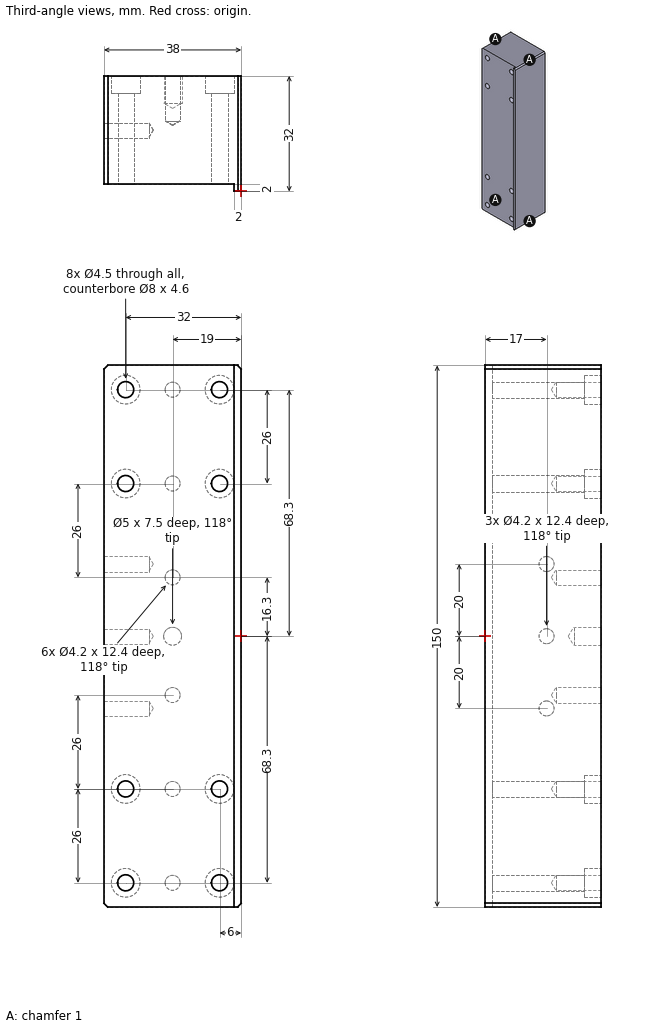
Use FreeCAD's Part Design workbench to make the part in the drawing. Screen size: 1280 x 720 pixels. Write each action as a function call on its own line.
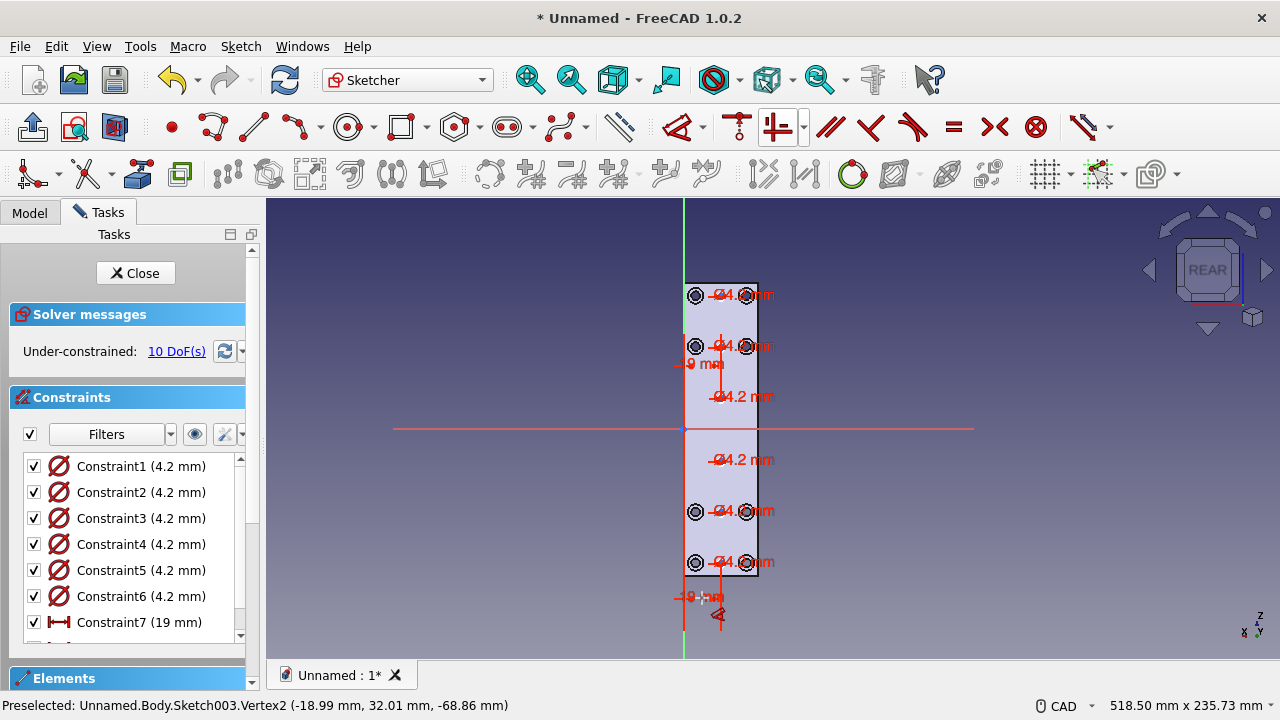
click(721, 513)
click(702, 547)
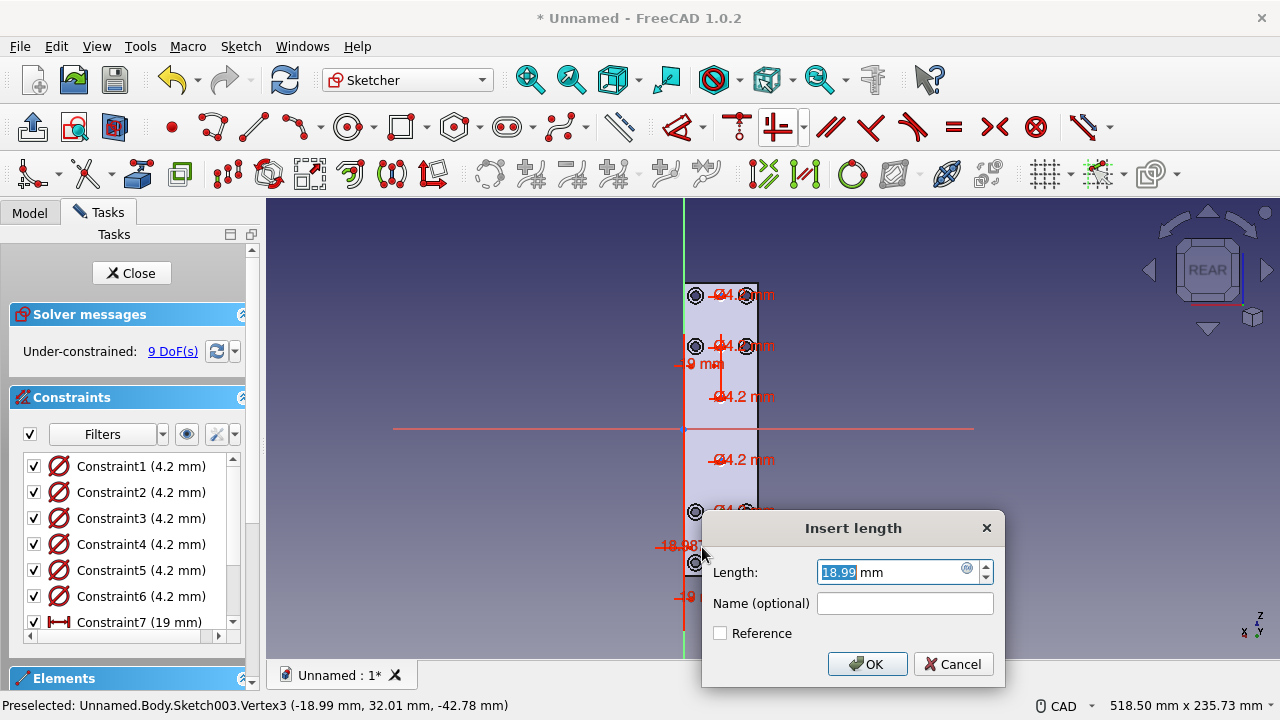
text(19)
key(Return)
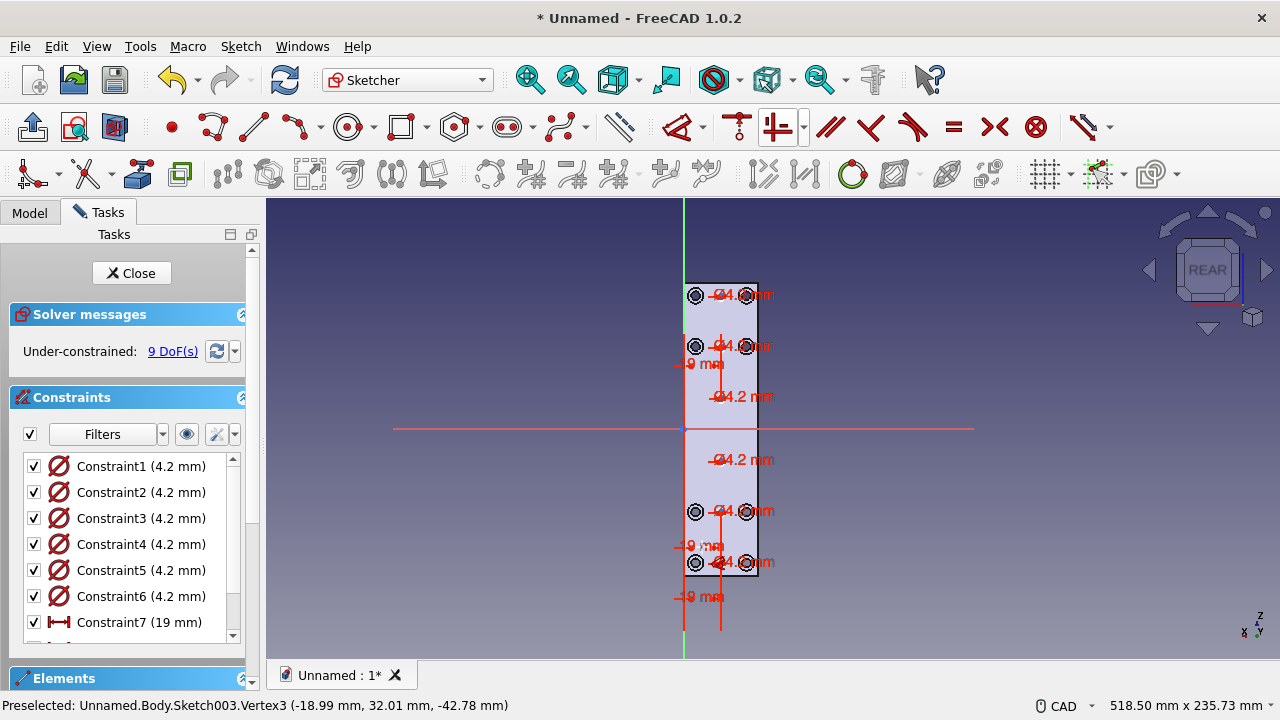
click(721, 348)
click(702, 314)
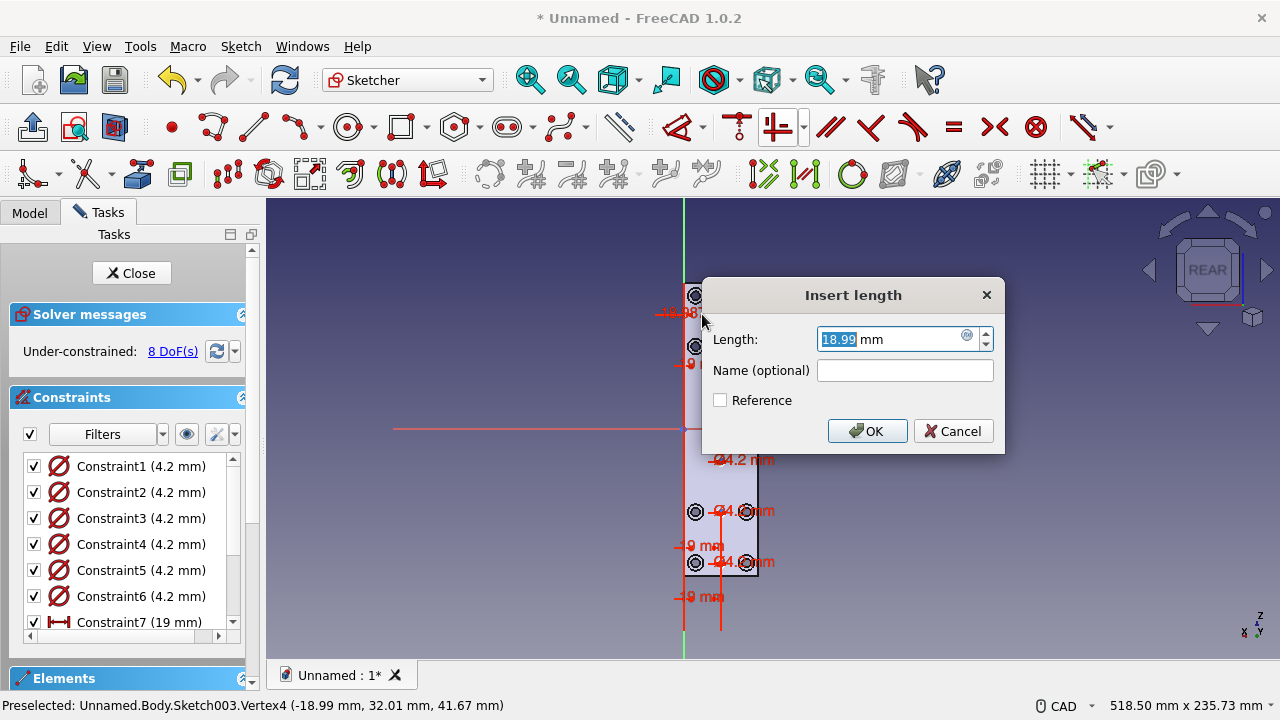
text(19)
key(Return)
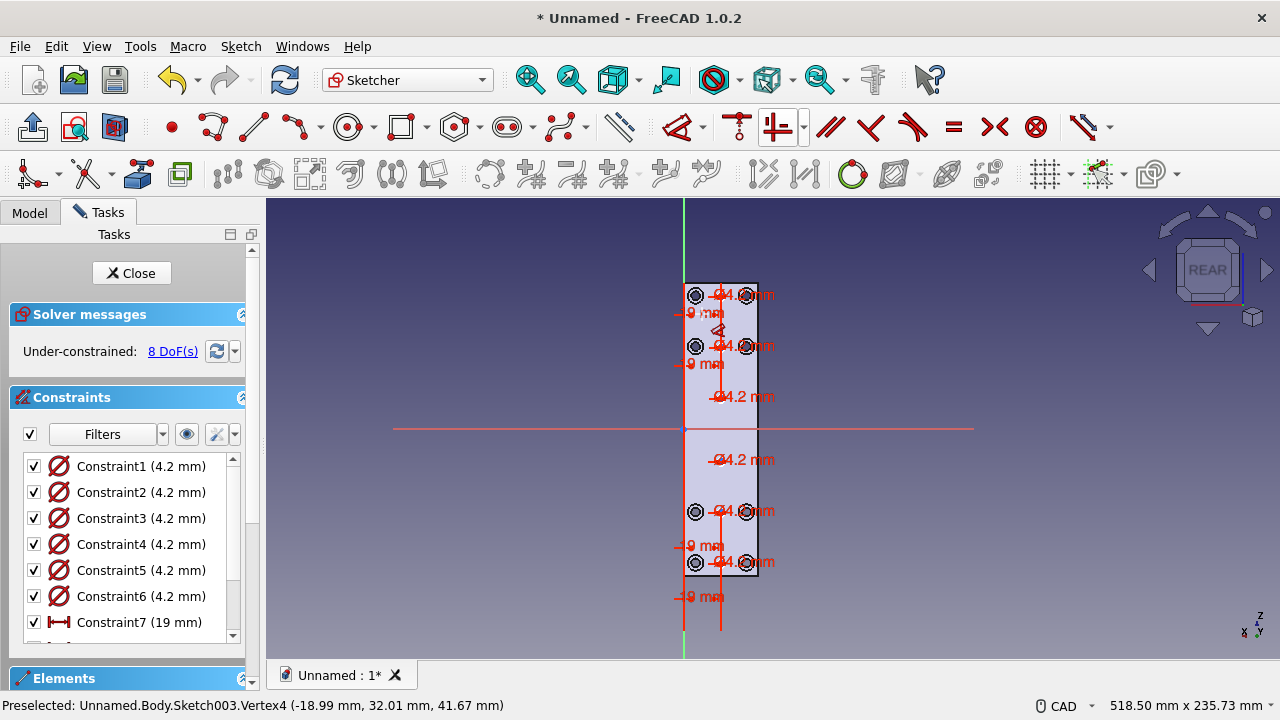
click(721, 297)
click(702, 263)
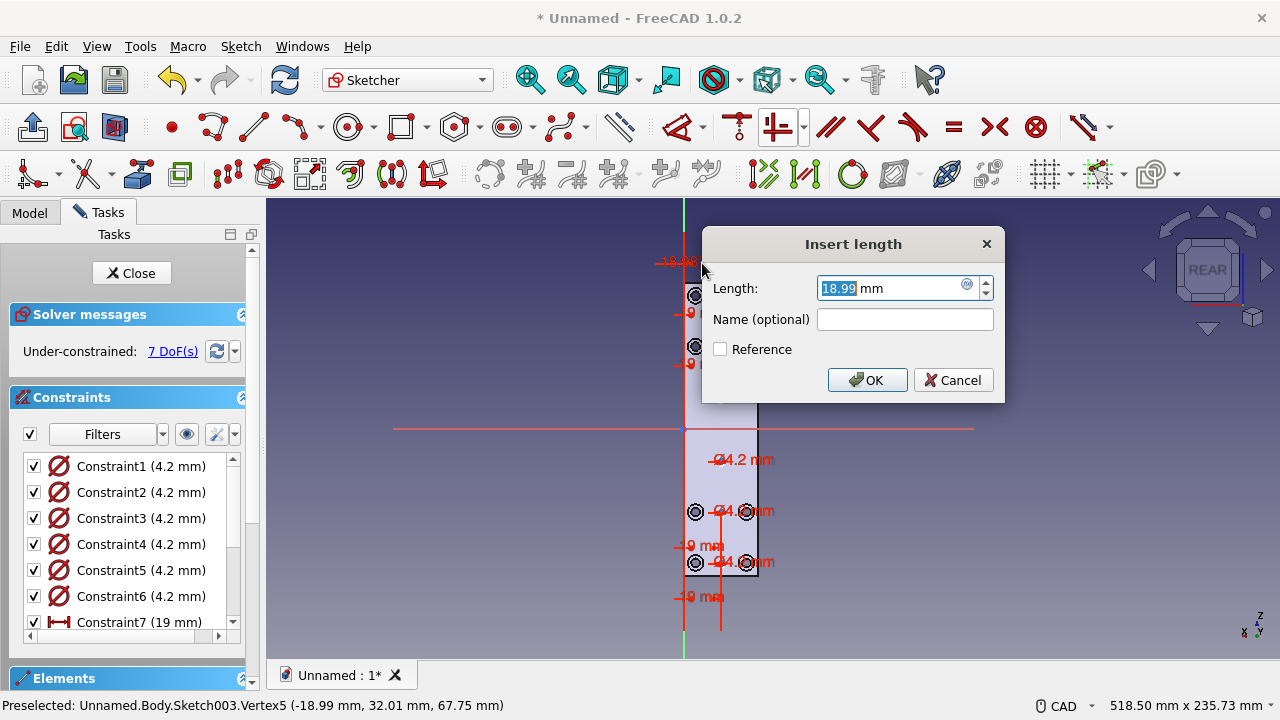
text(19)
key(Return)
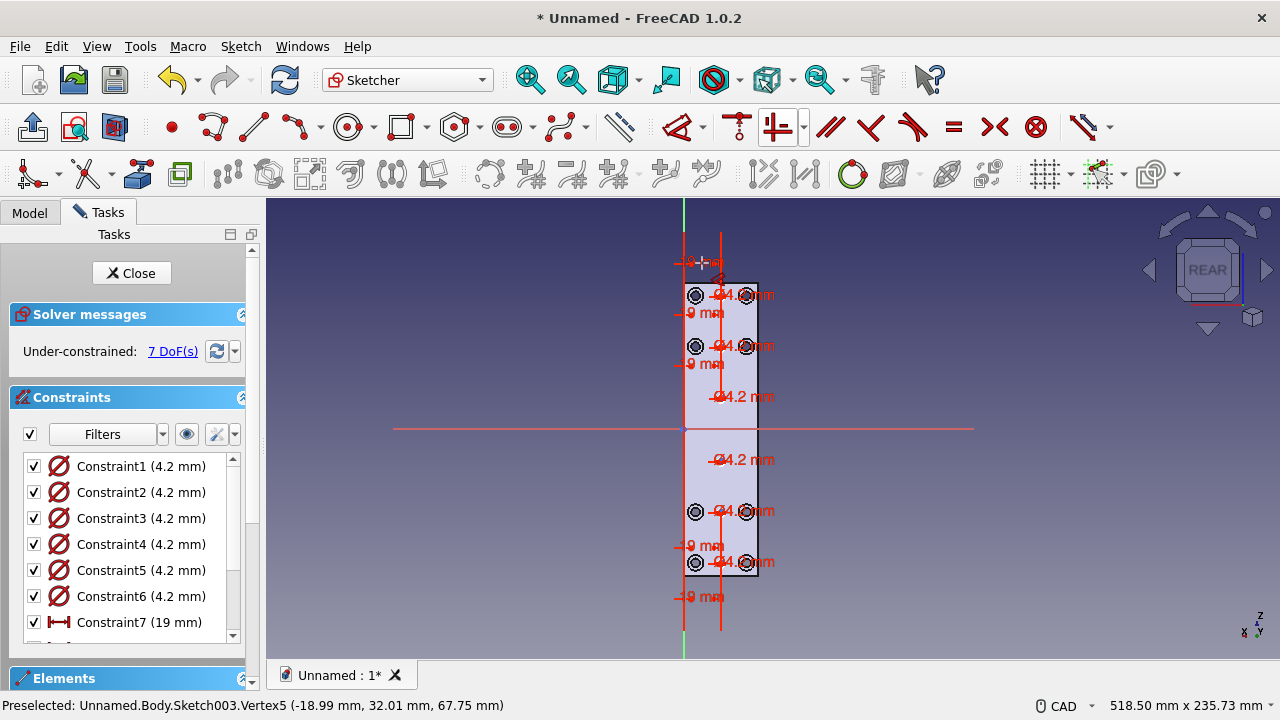
click(721, 462)
click(702, 496)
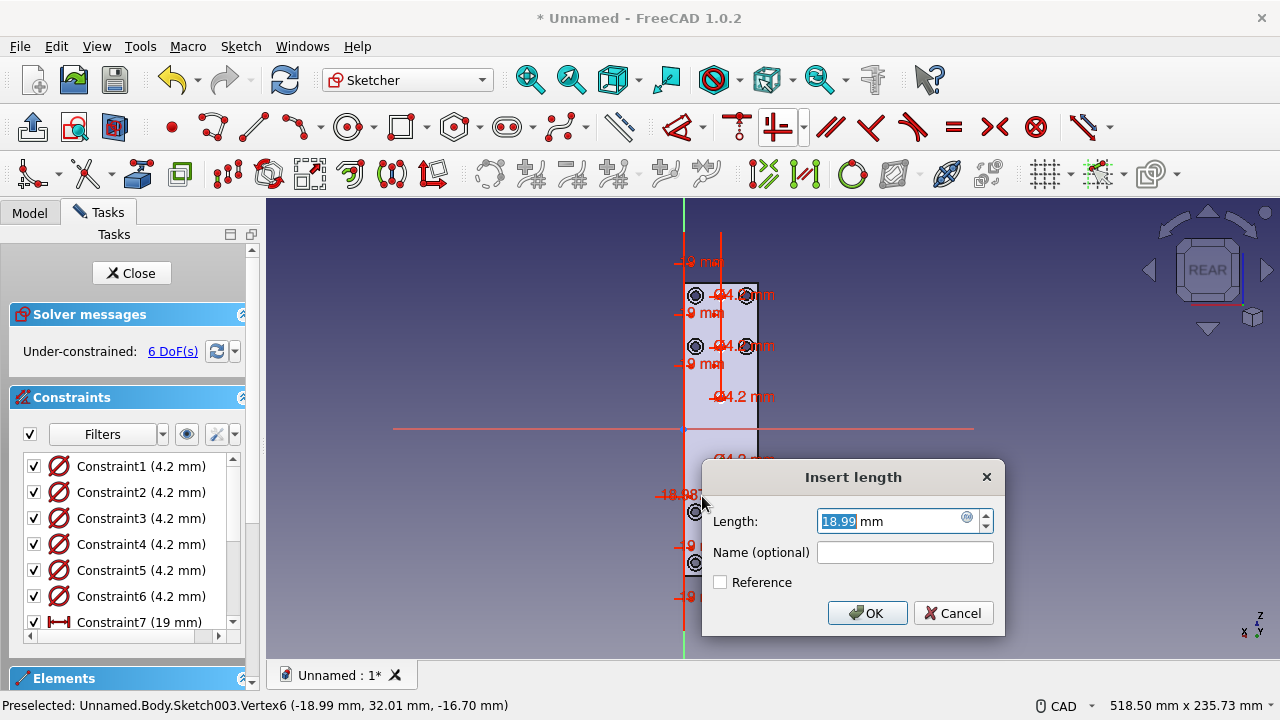
text(19)
key(Return)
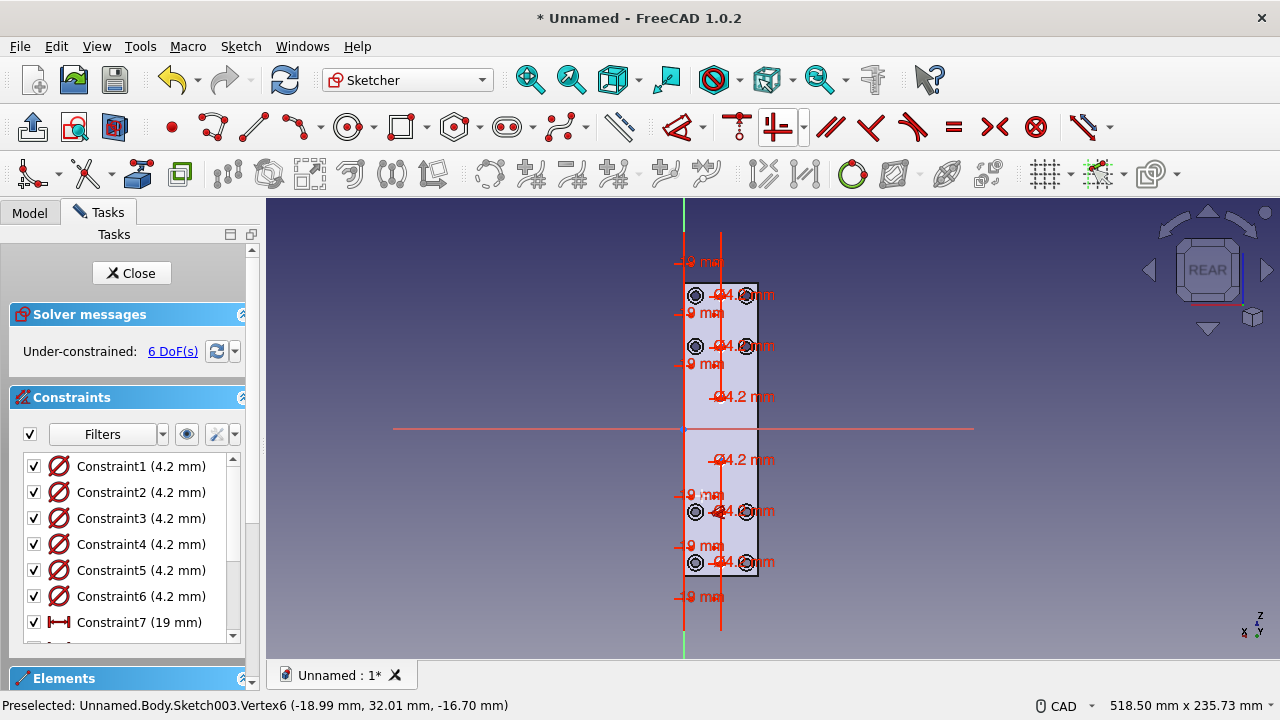
click(721, 564)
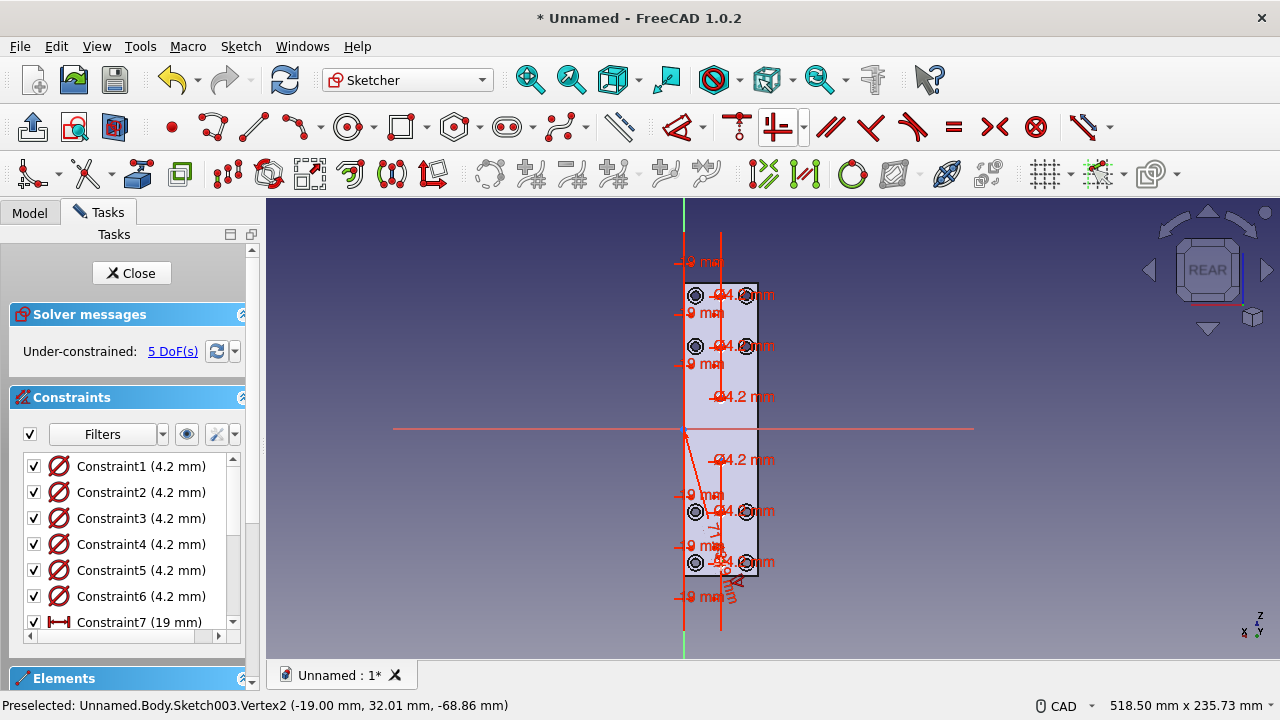
click(721, 513)
click(755, 527)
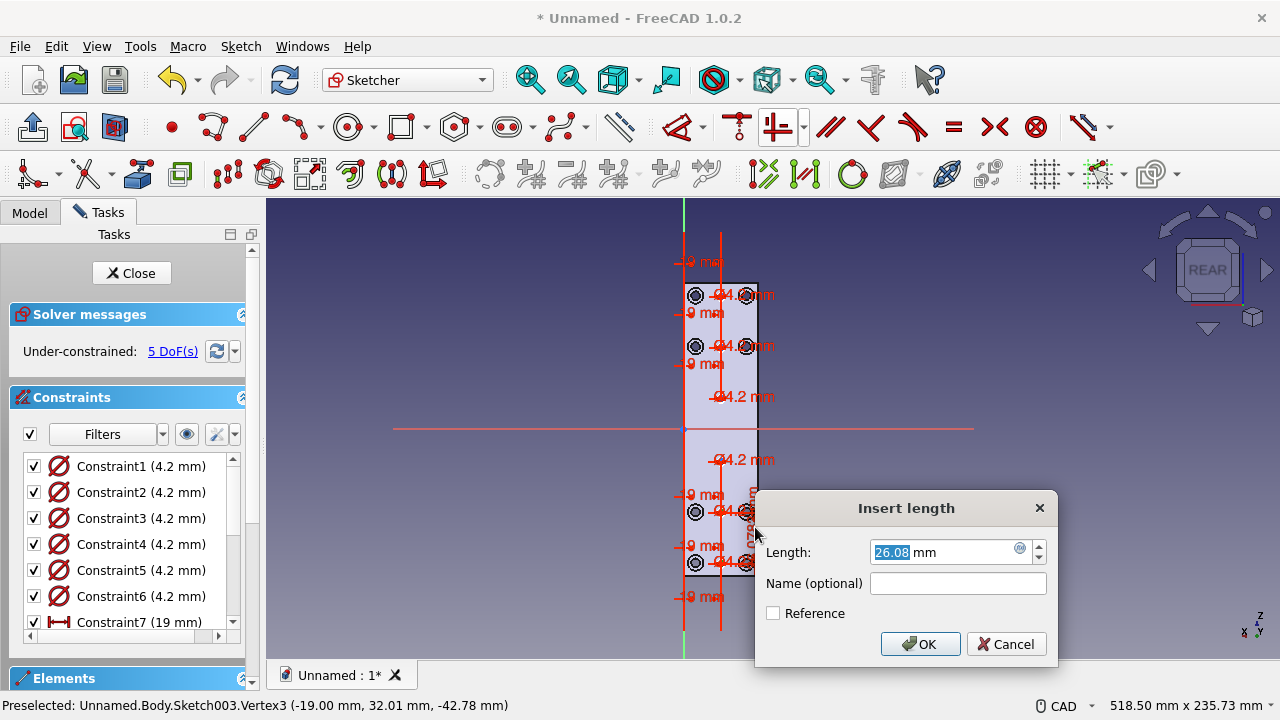
text(26)
key(Return)